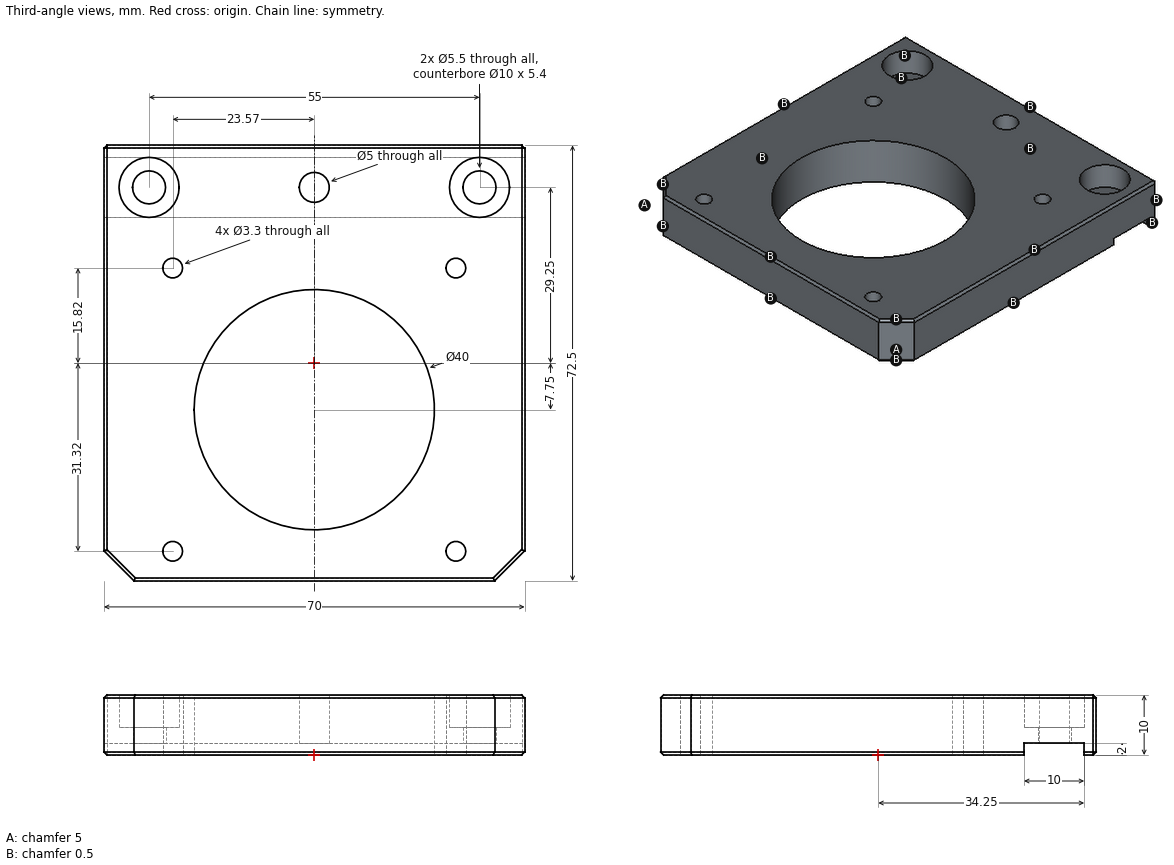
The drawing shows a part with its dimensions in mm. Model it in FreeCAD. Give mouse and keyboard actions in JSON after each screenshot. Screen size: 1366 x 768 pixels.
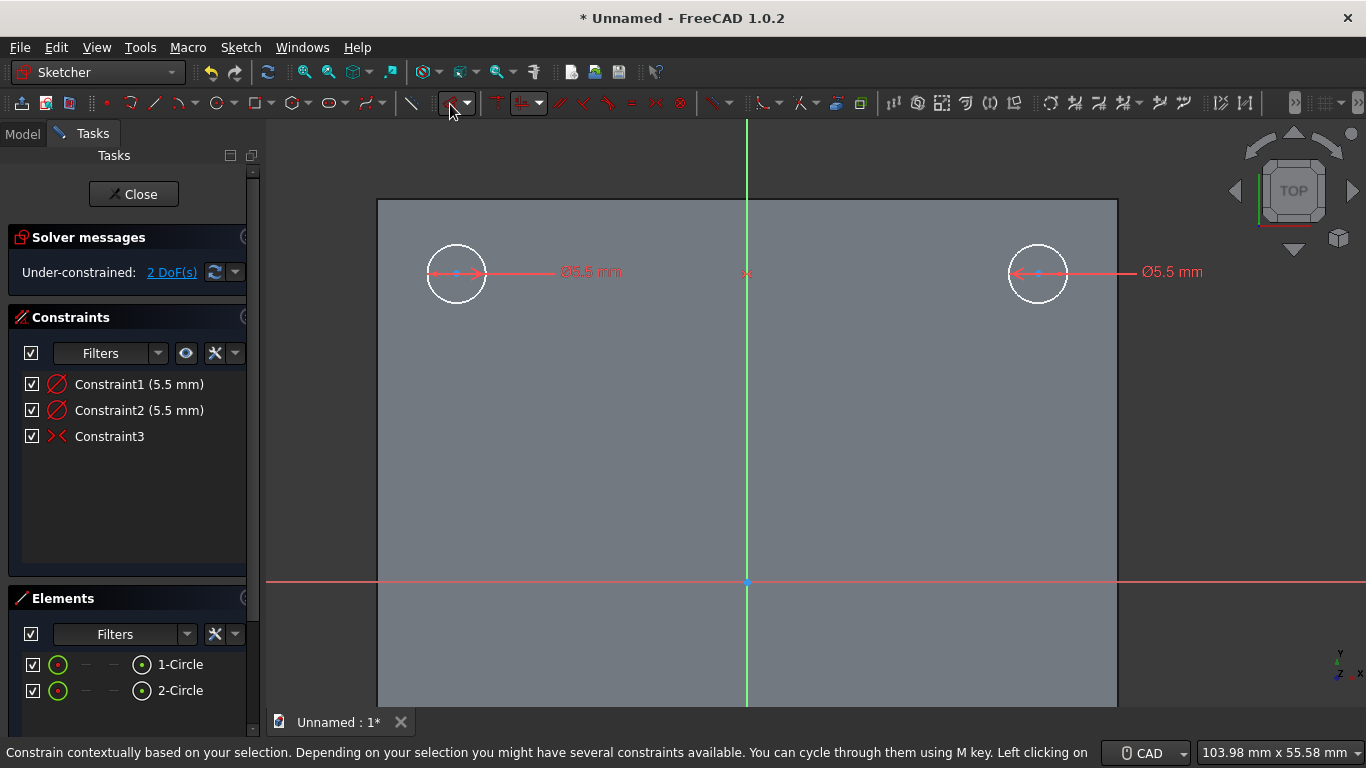
{"action": "left_click", "coordinate": [1038, 274]}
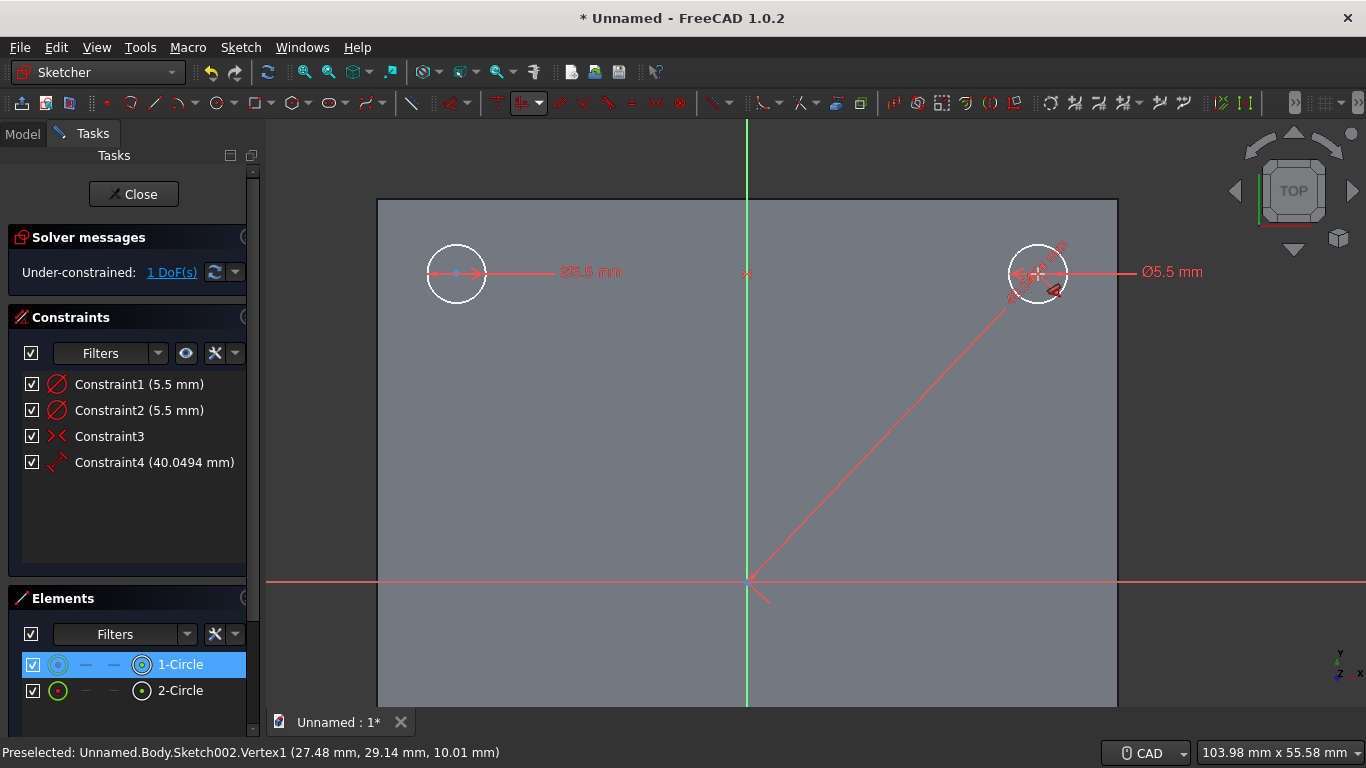
{"action": "left_click", "coordinate": [457, 274]}
{"action": "left_click", "coordinate": [614, 240]}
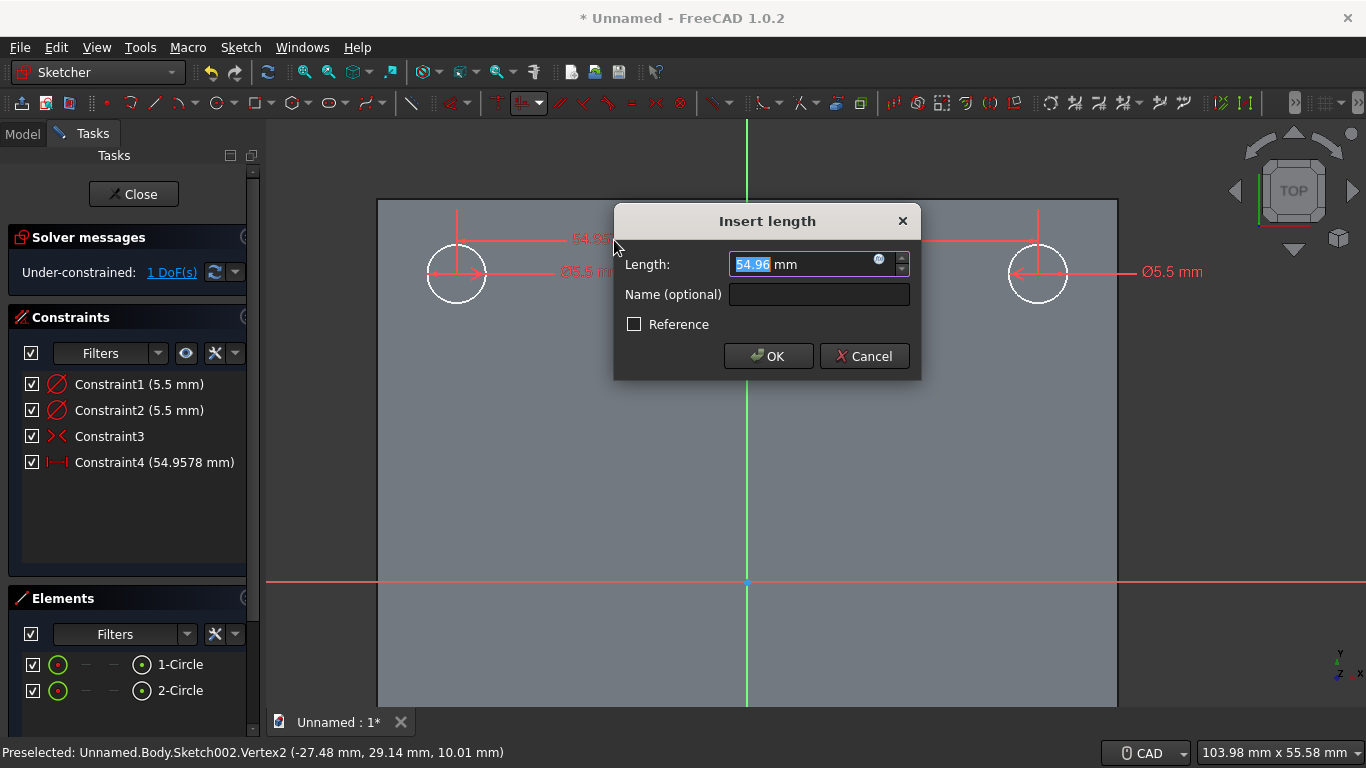
{"action": "type", "text": "55"}
{"action": "key", "text": "Return"}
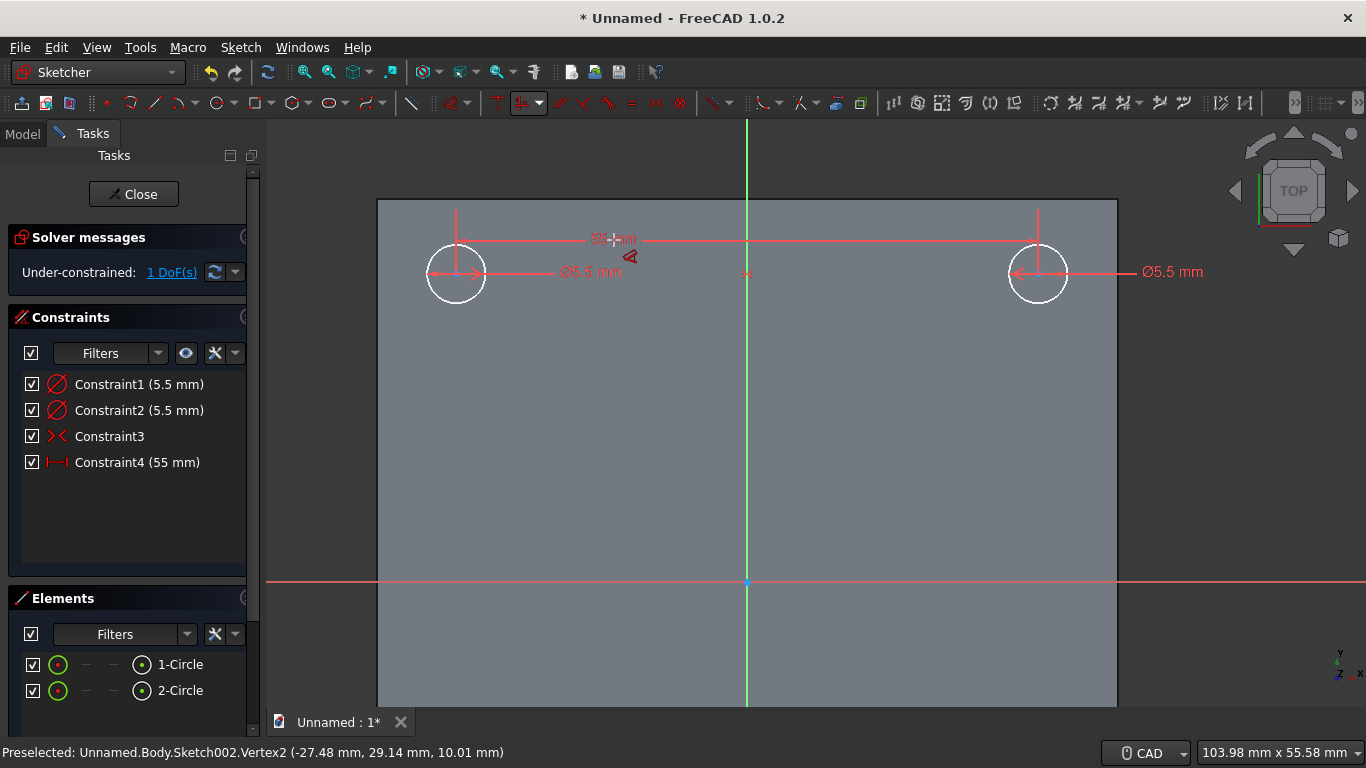
{"action": "left_click", "coordinate": [1038, 274]}
{"action": "left_click", "coordinate": [1072, 428]}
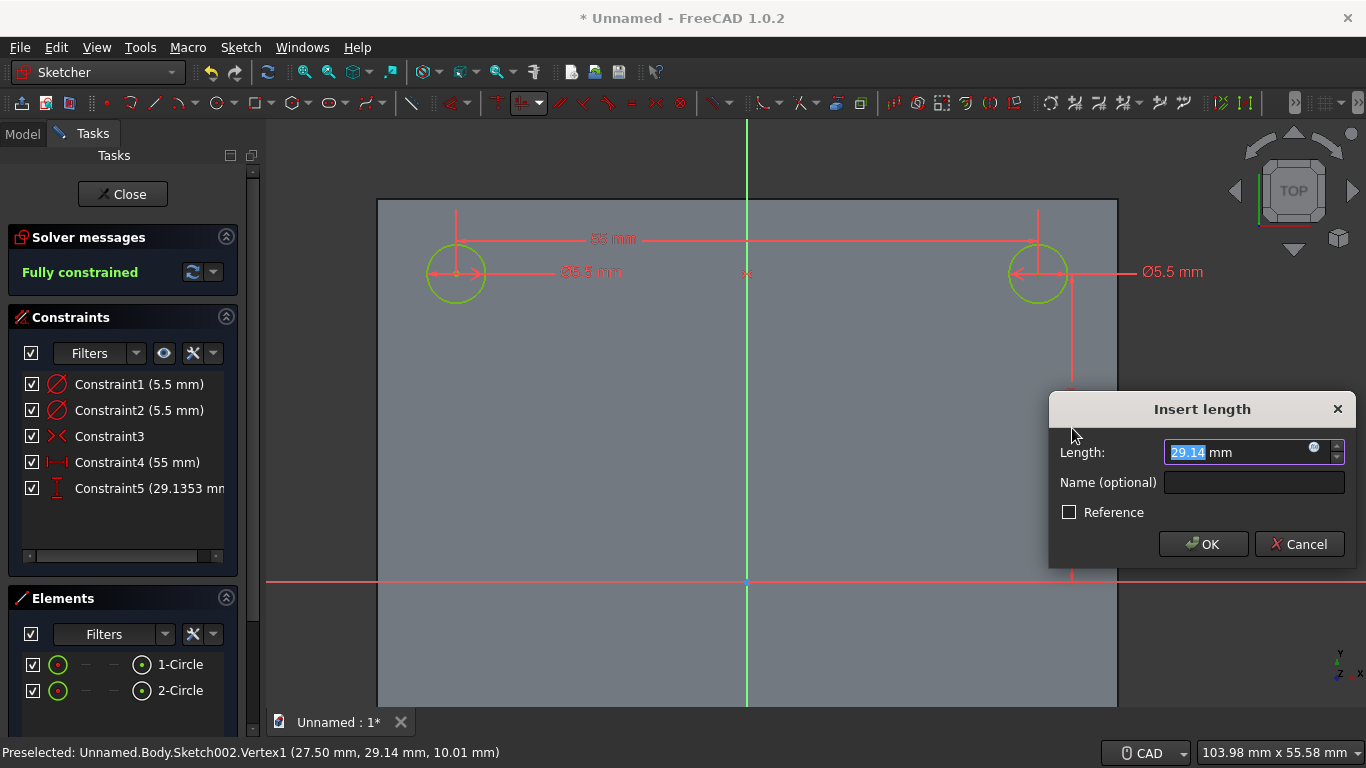
{"action": "type", "text": "29.25"}
{"action": "key", "text": "Return"}
{"action": "key", "text": "Escape"}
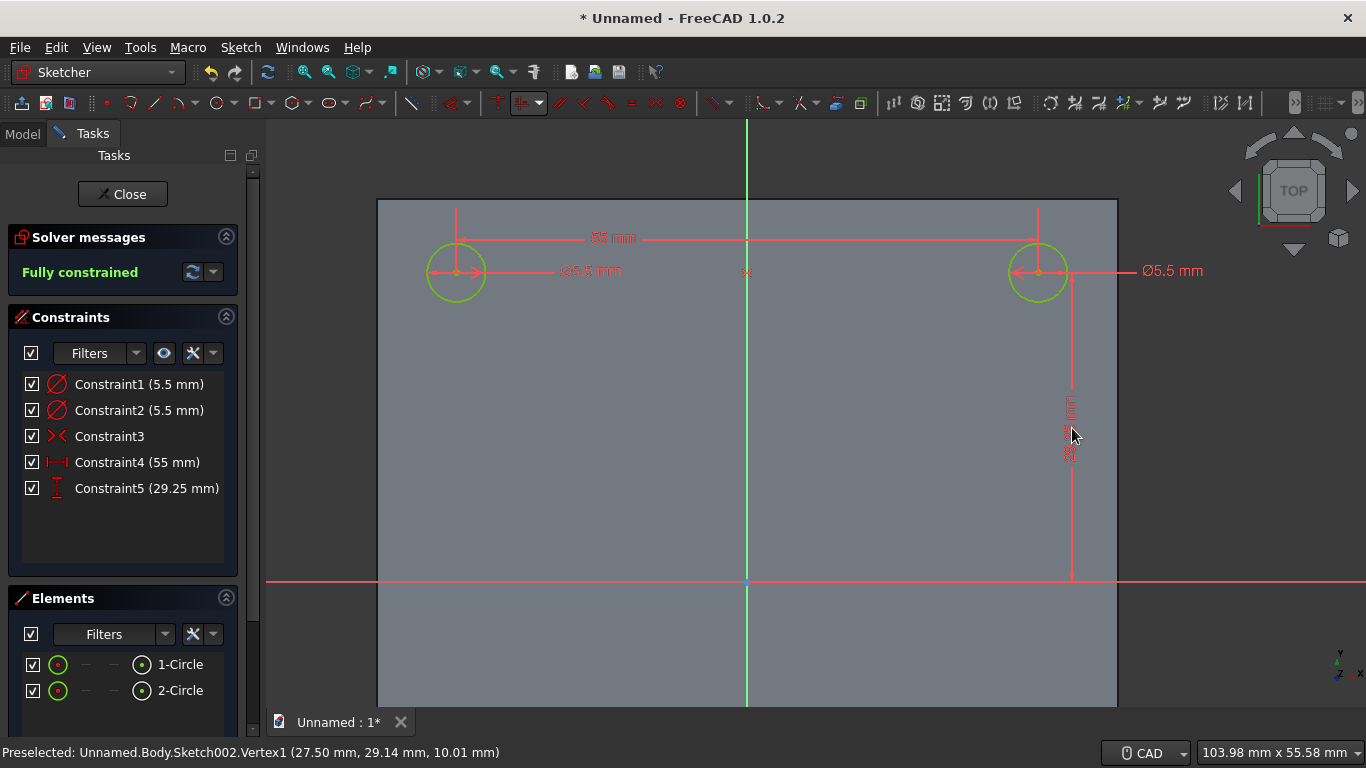
{"action": "left_click", "coordinate": [123, 194]}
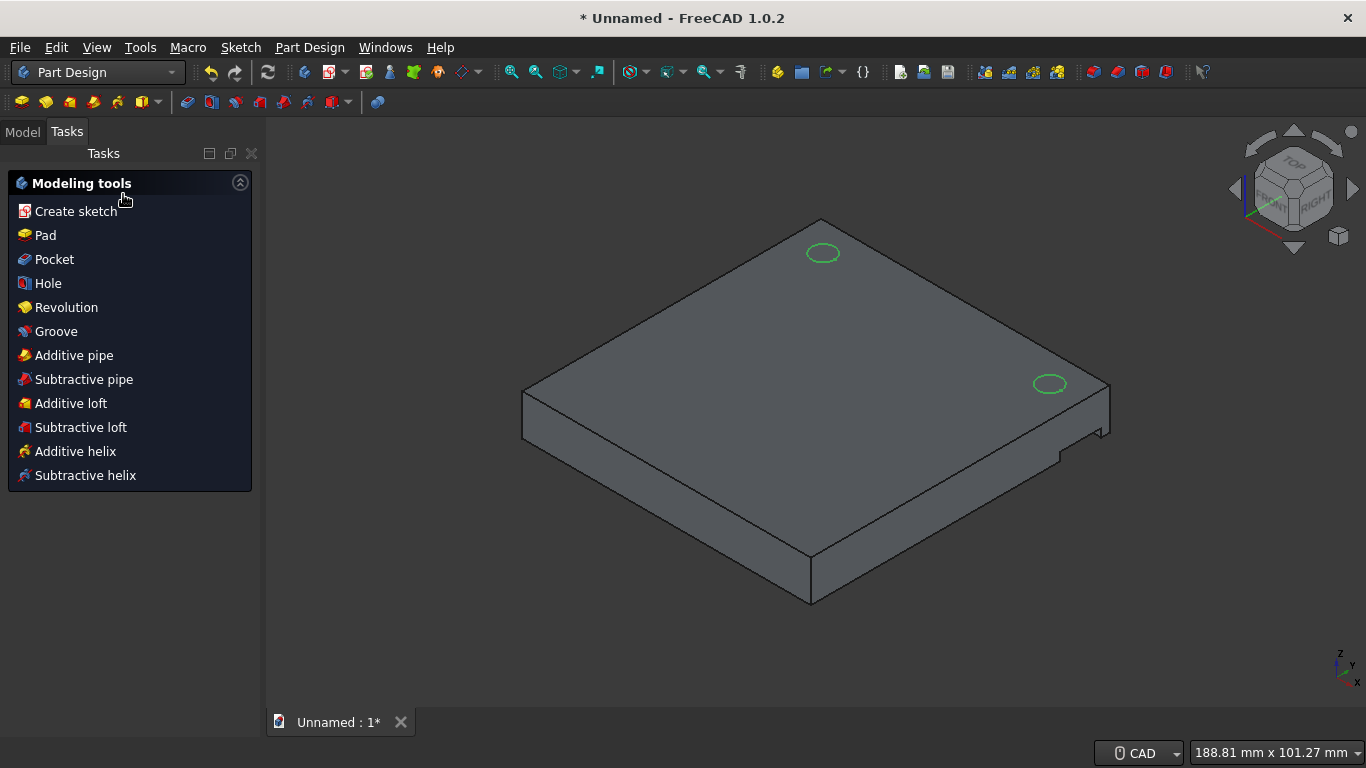
{"action": "left_click", "coordinate": [212, 102]}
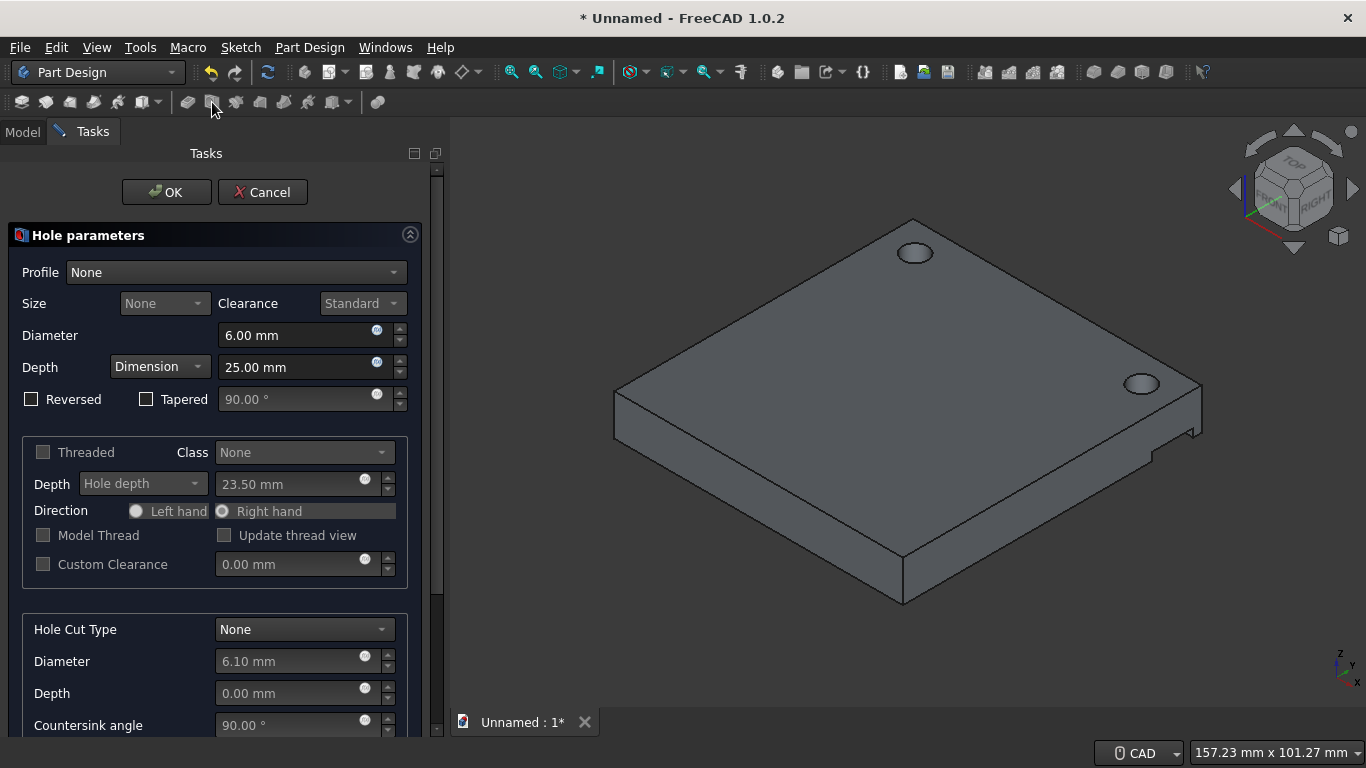
{"action": "triple_click", "coordinate": [305, 335]}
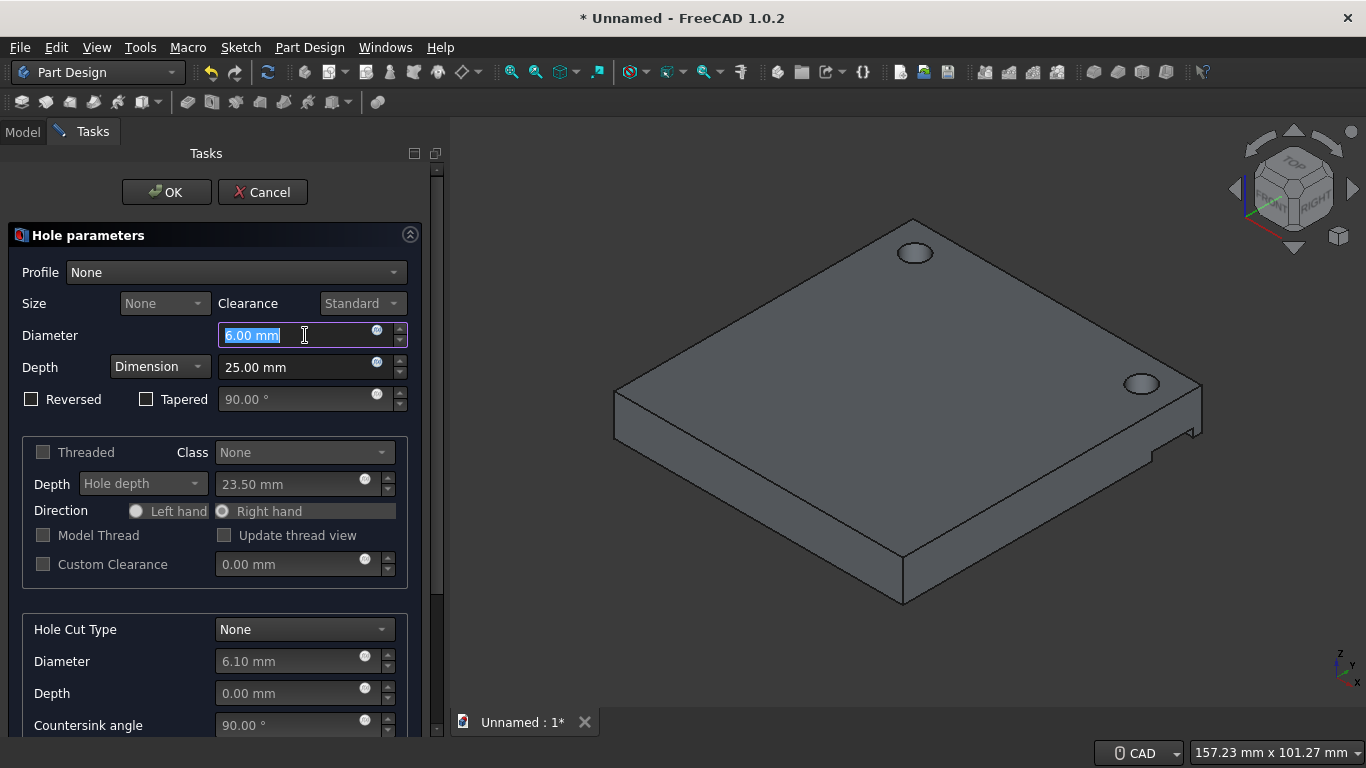
{"action": "type", "text": "5.5"}
{"action": "key", "text": "Tab"}